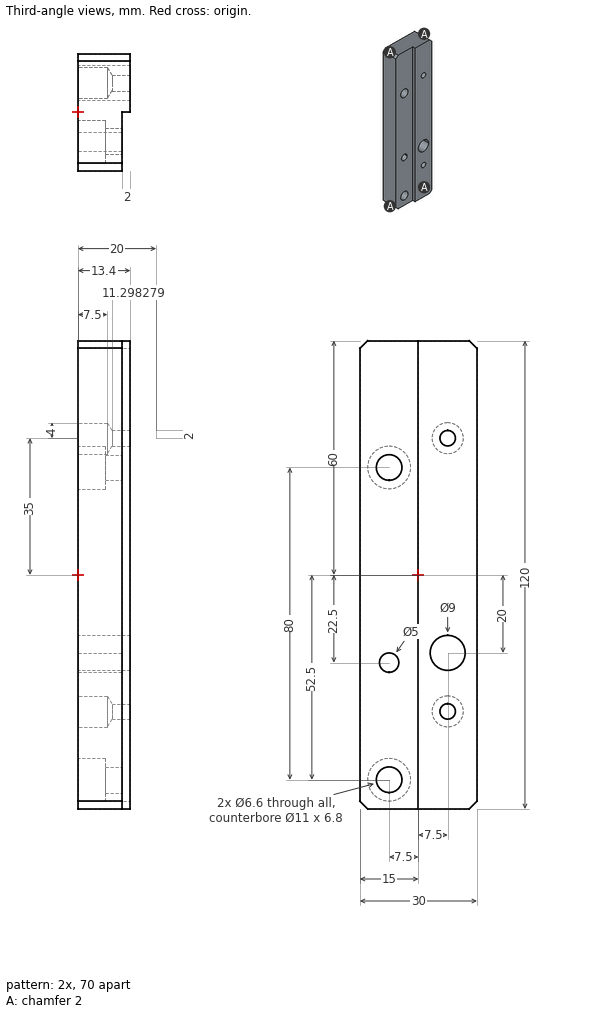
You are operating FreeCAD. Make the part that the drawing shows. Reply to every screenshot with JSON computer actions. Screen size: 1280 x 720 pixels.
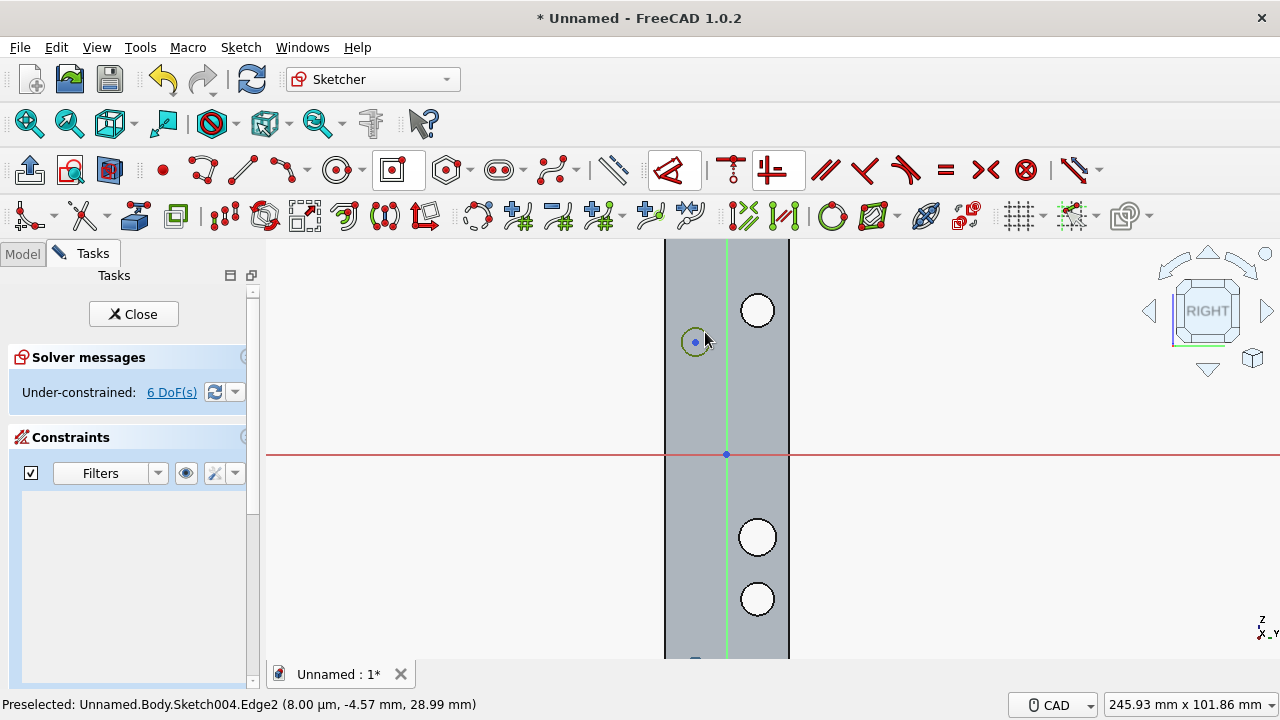
{"action": "left_click", "coordinate": [946, 170]}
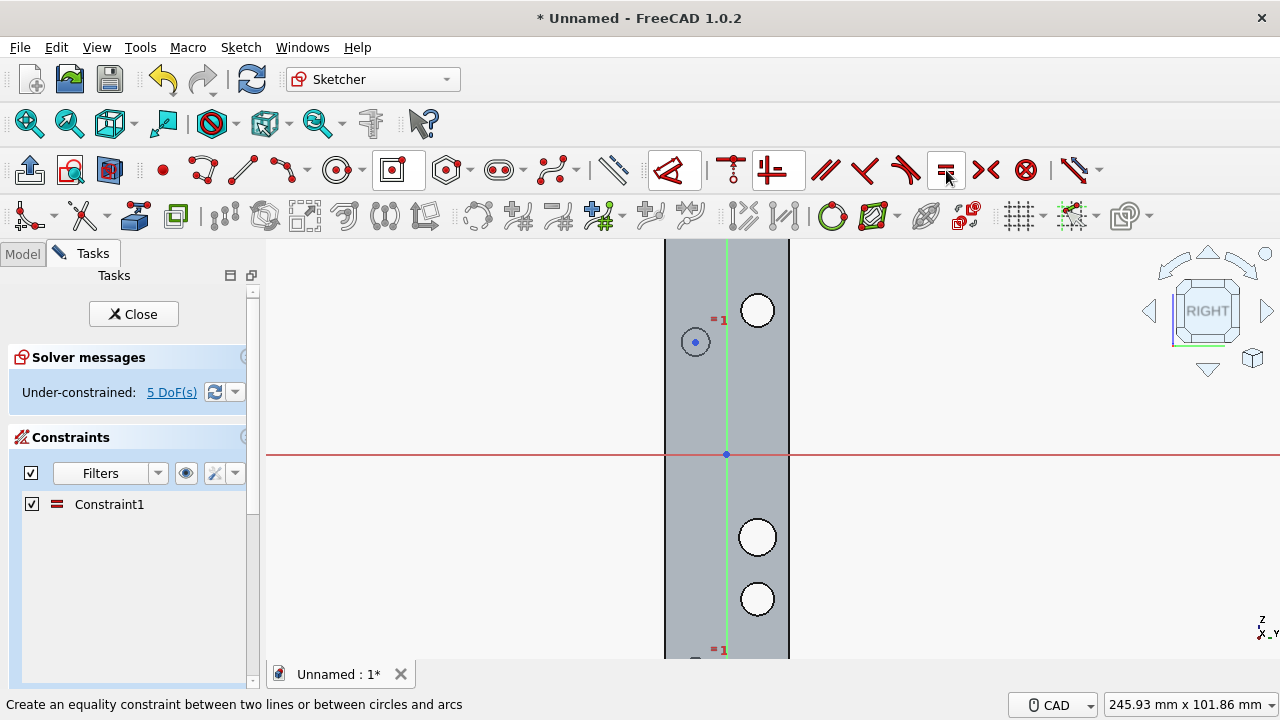
{"action": "scroll", "coordinate": [705, 332], "scroll_direction": "down", "scroll_amount": 2}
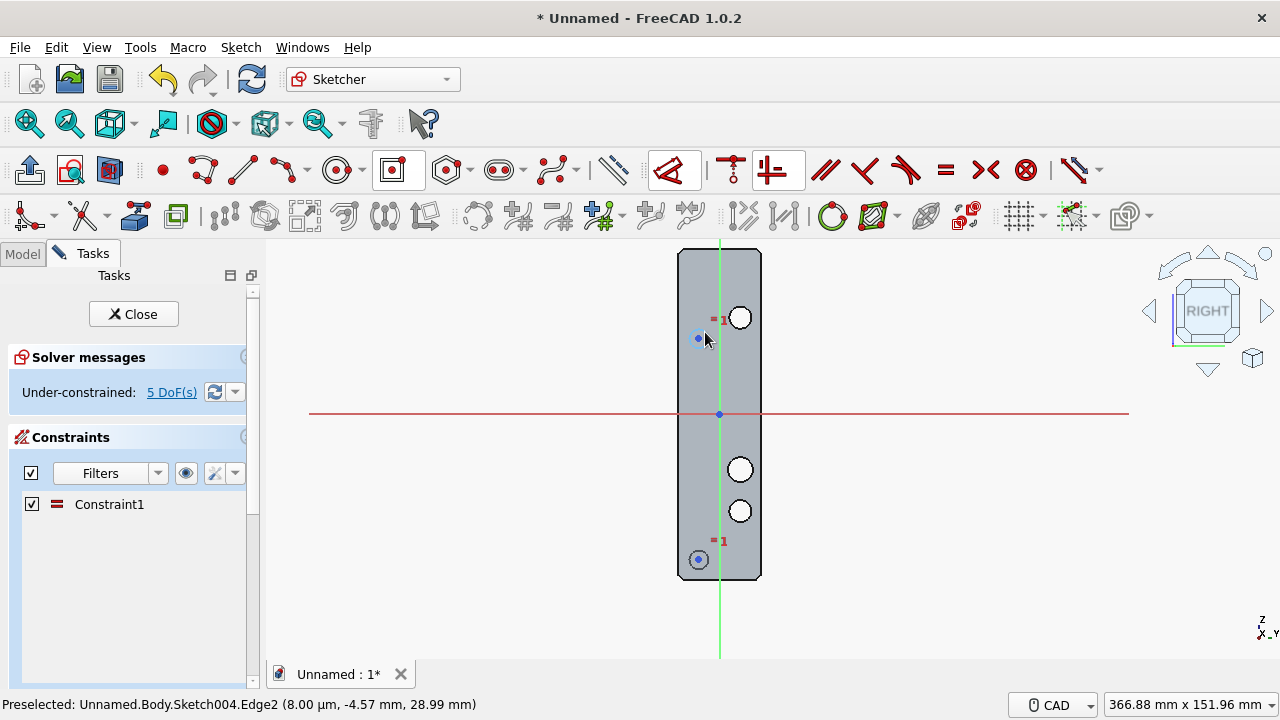
{"action": "left_click", "coordinate": [699, 560]}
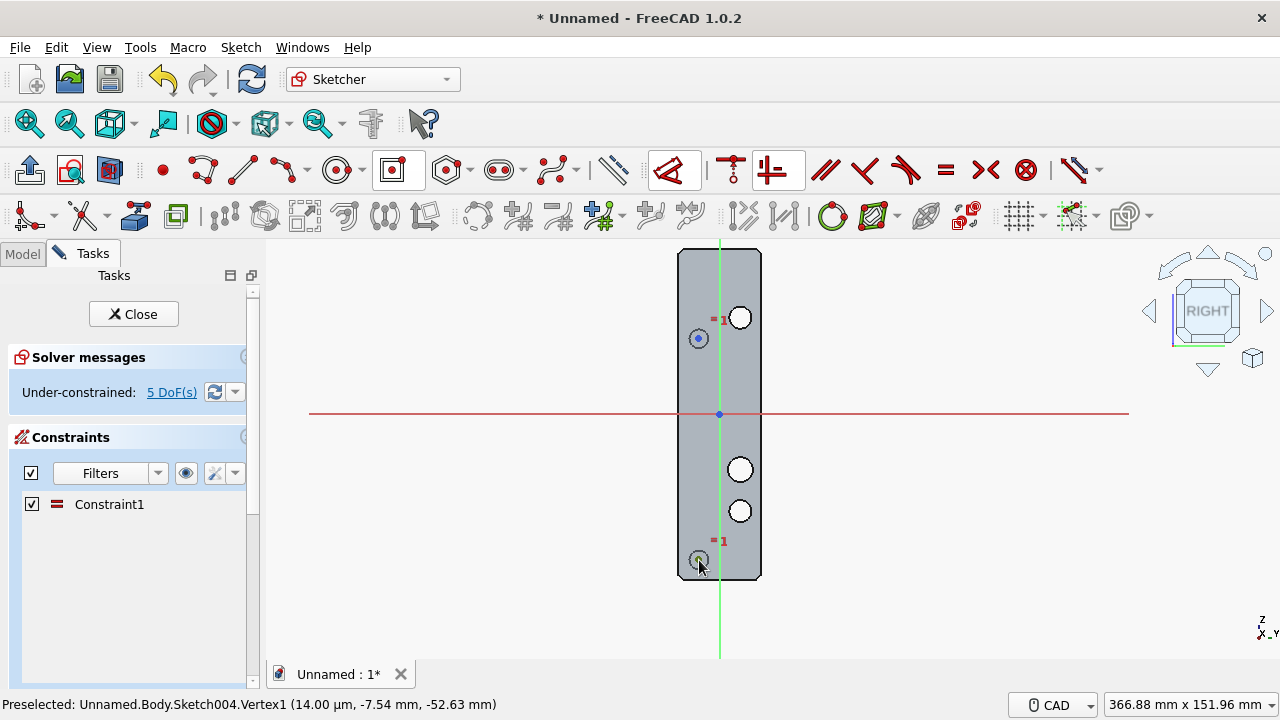
{"action": "left_click", "coordinate": [699, 339]}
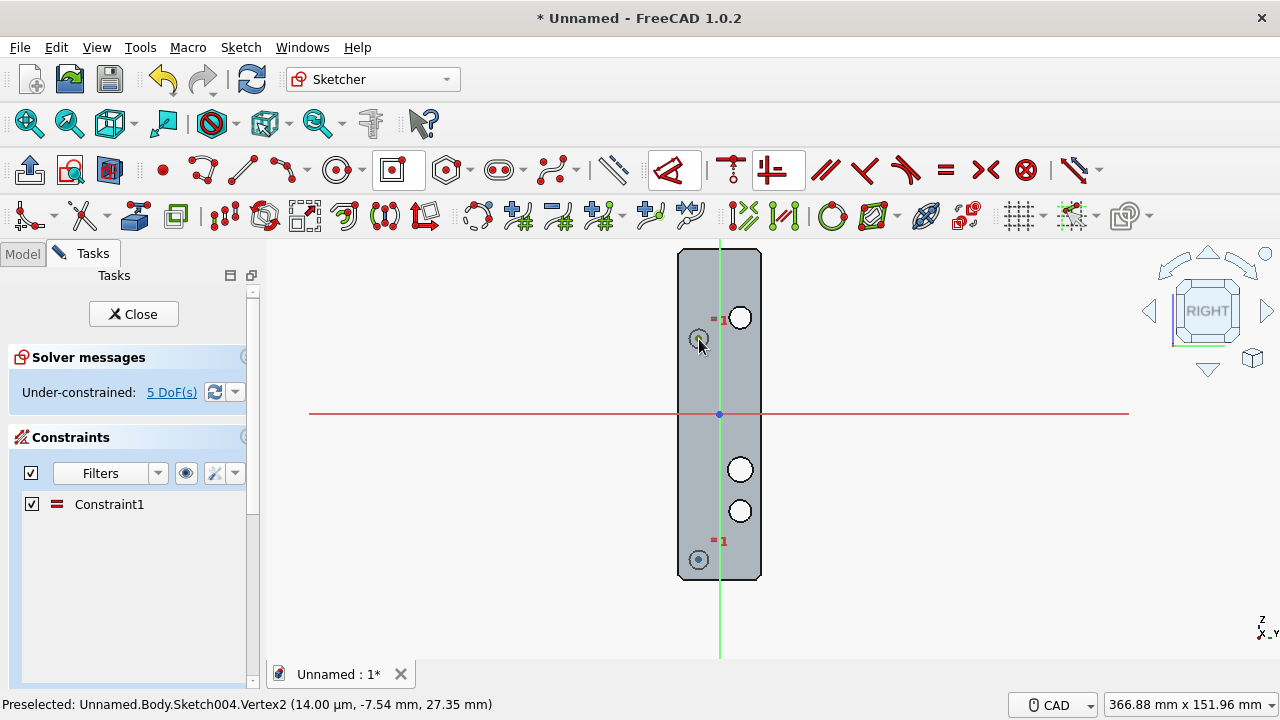
{"action": "key", "text": "v"}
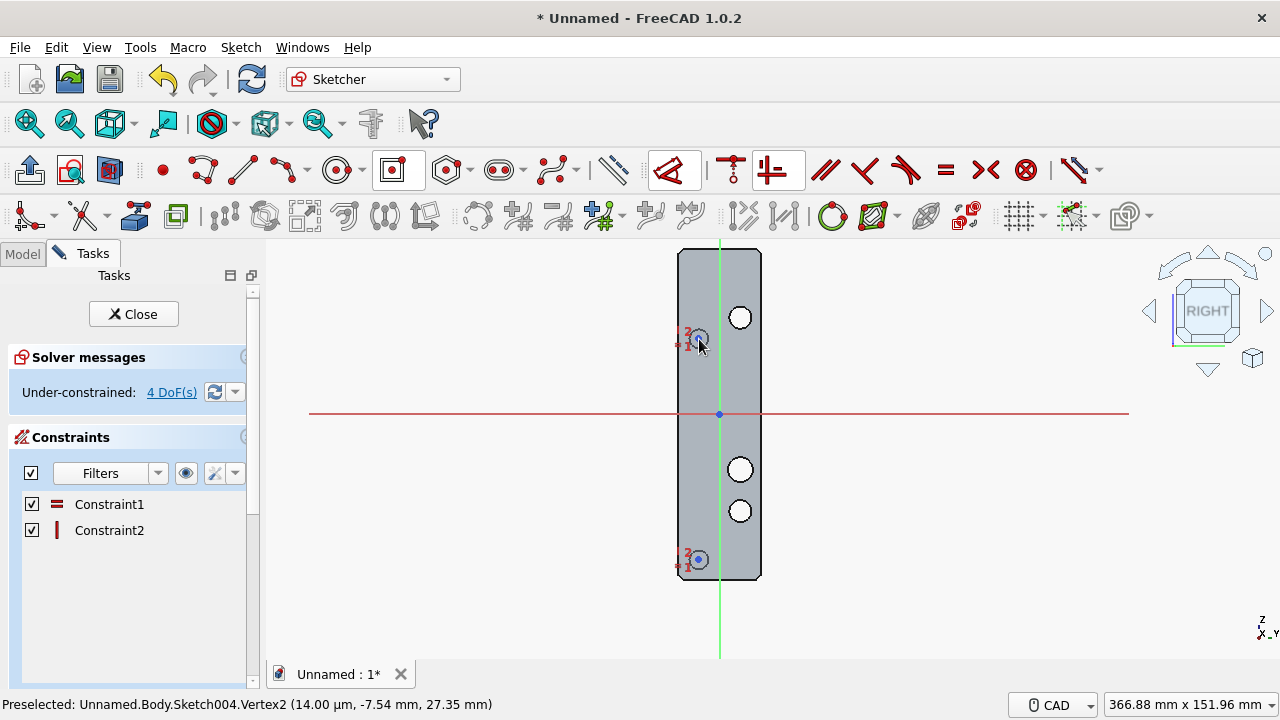
{"action": "scroll", "coordinate": [705, 553], "scroll_direction": "up", "scroll_amount": 4}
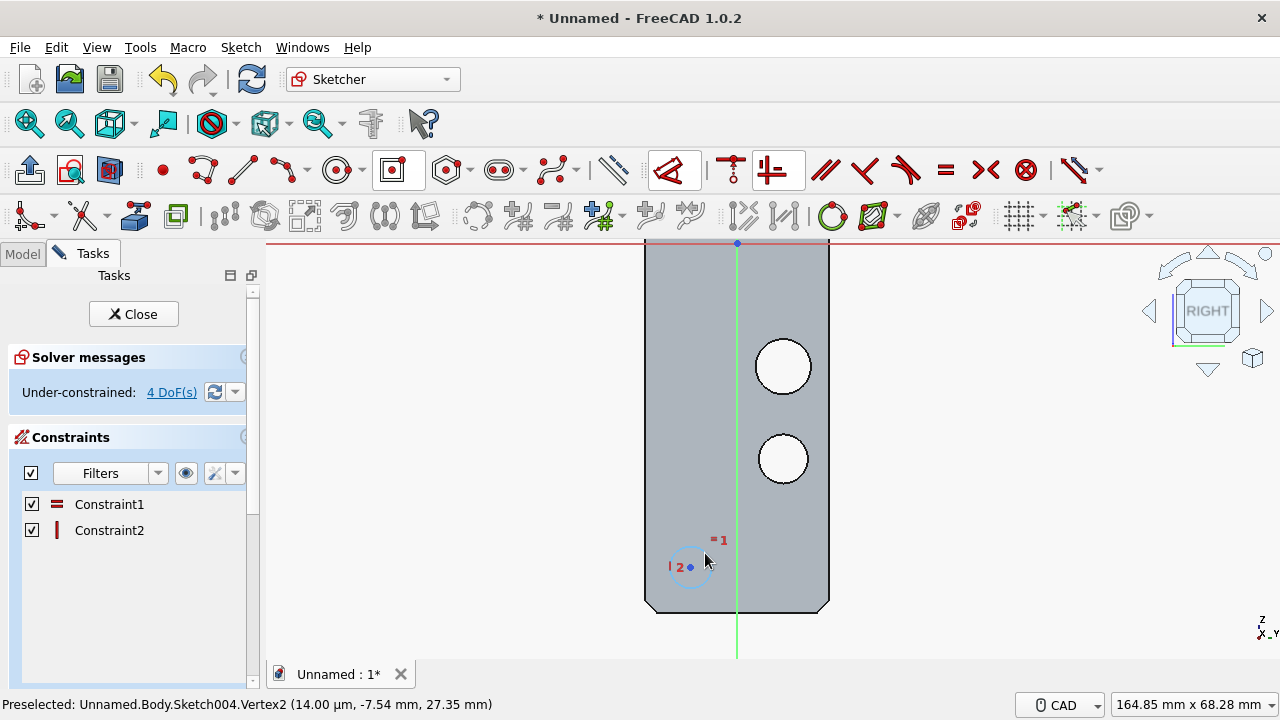
{"action": "left_click", "coordinate": [706, 553]}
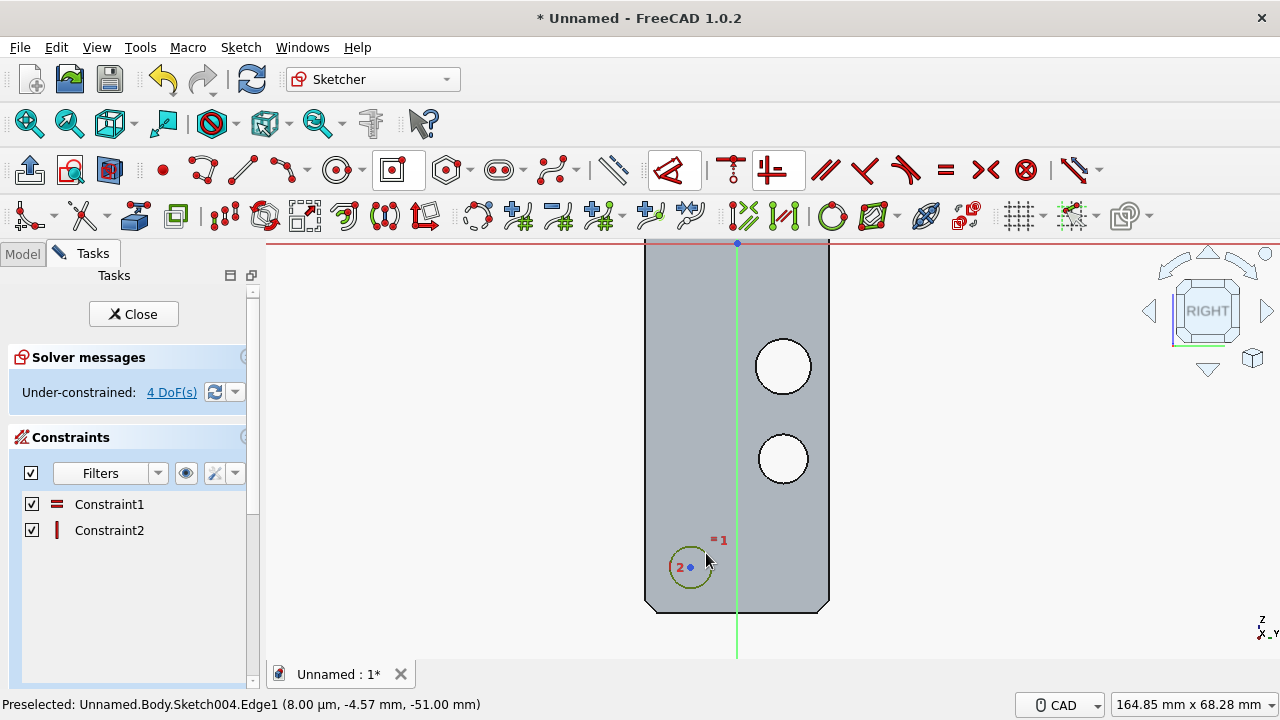
{"action": "key", "text": "k o"}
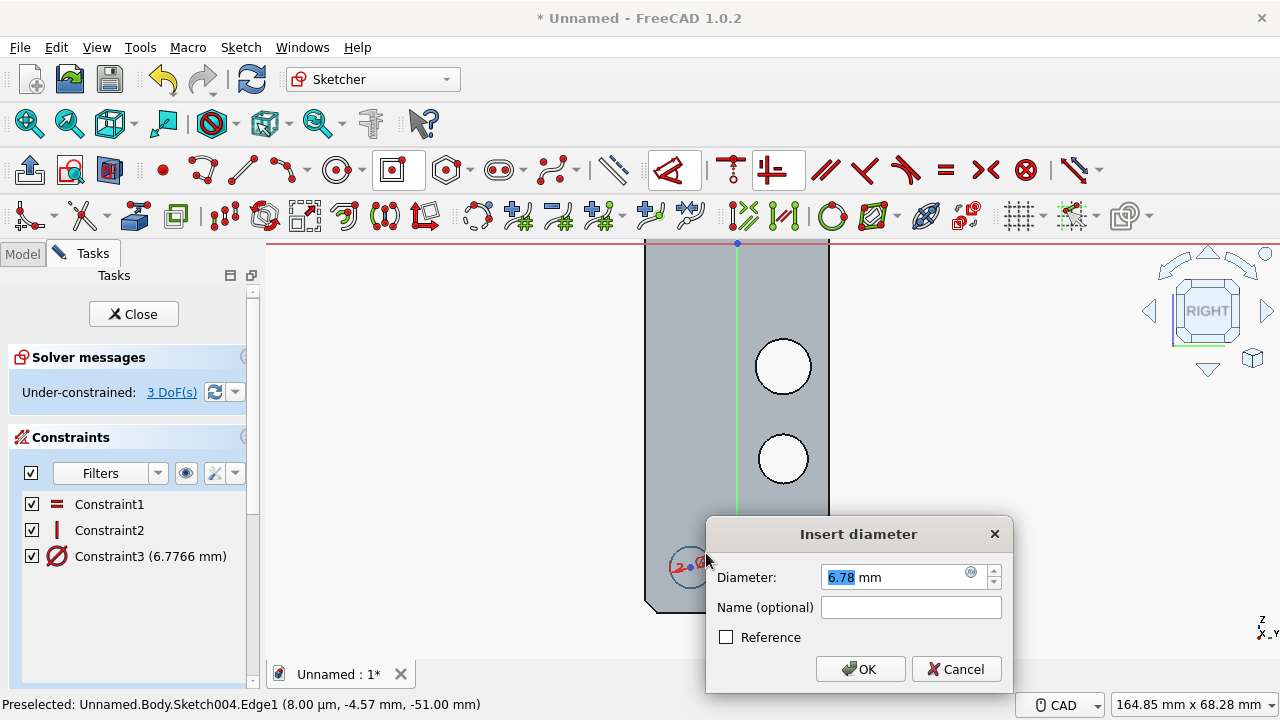
{"action": "type", "text": "6.6"}
{"action": "key", "text": "Return"}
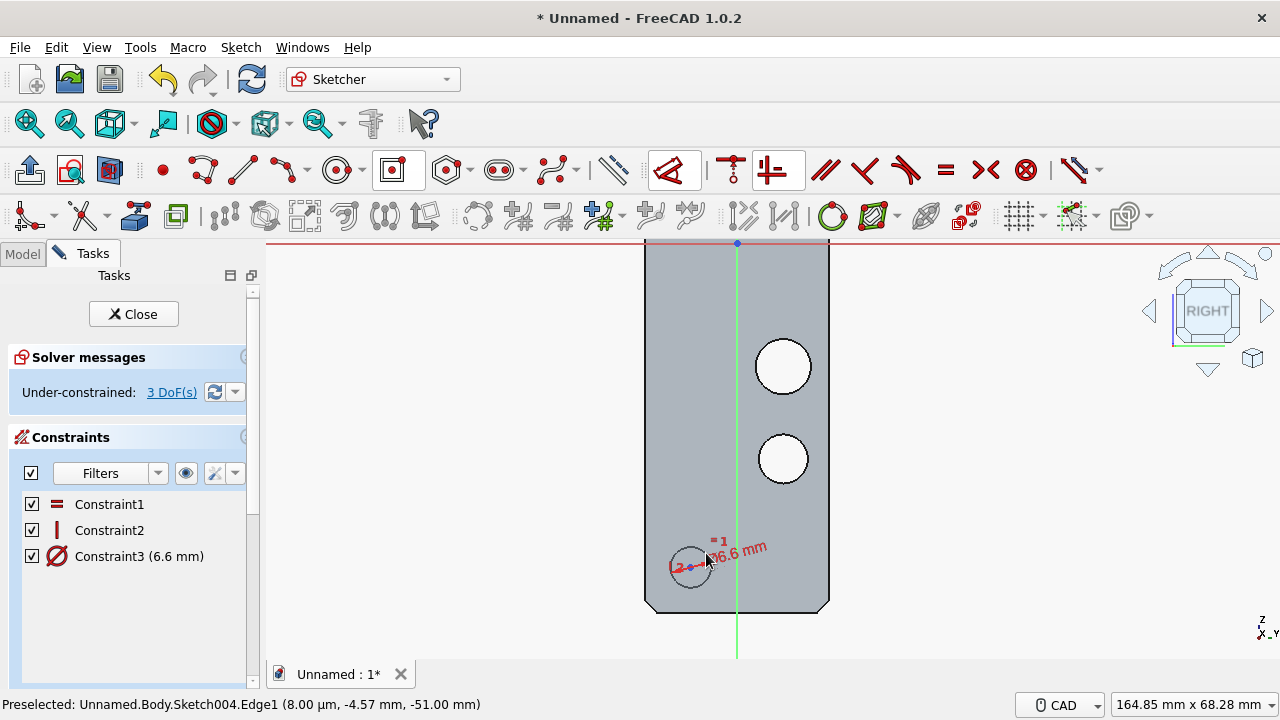
{"action": "left_click", "coordinate": [691, 567]}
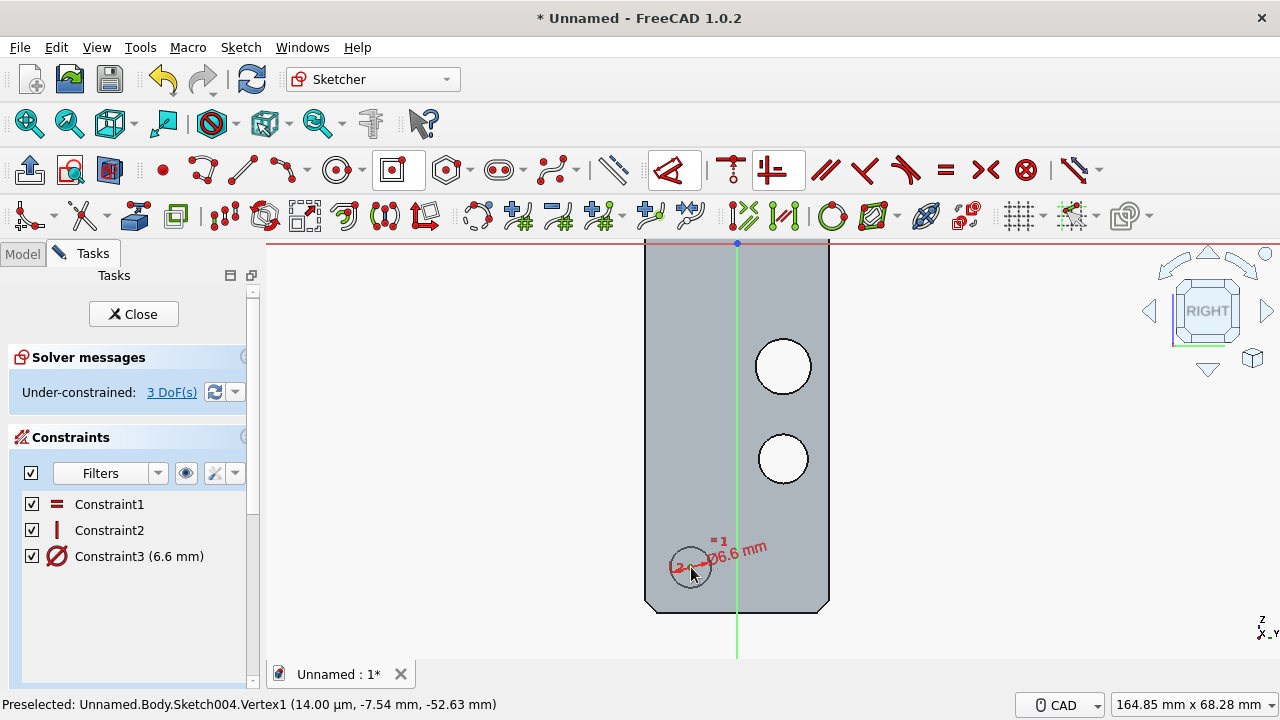
{"action": "left_click", "coordinate": [696, 170]}